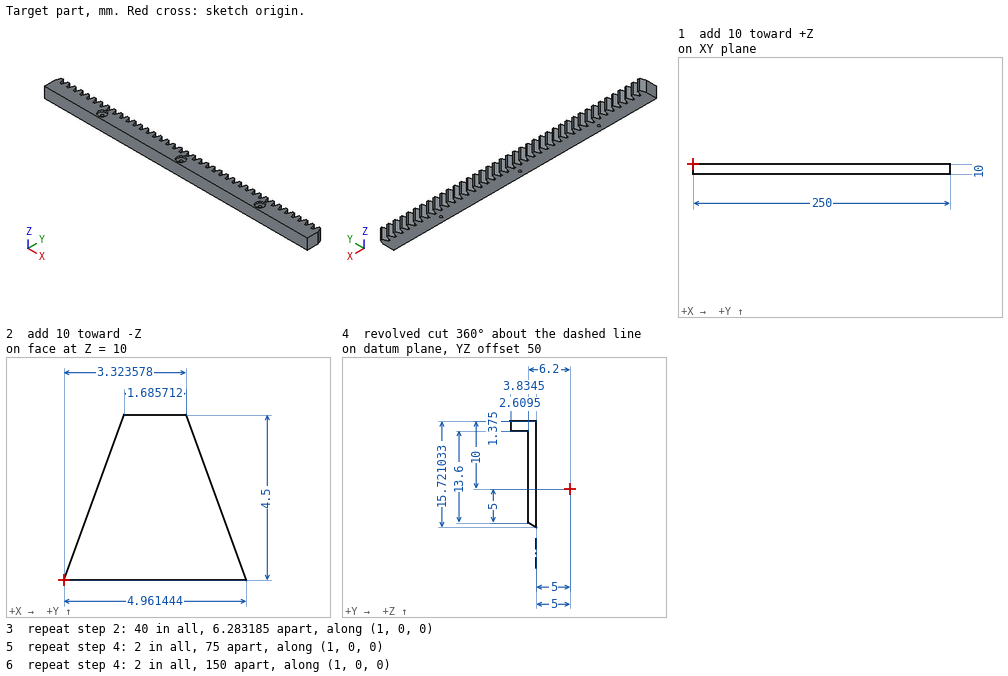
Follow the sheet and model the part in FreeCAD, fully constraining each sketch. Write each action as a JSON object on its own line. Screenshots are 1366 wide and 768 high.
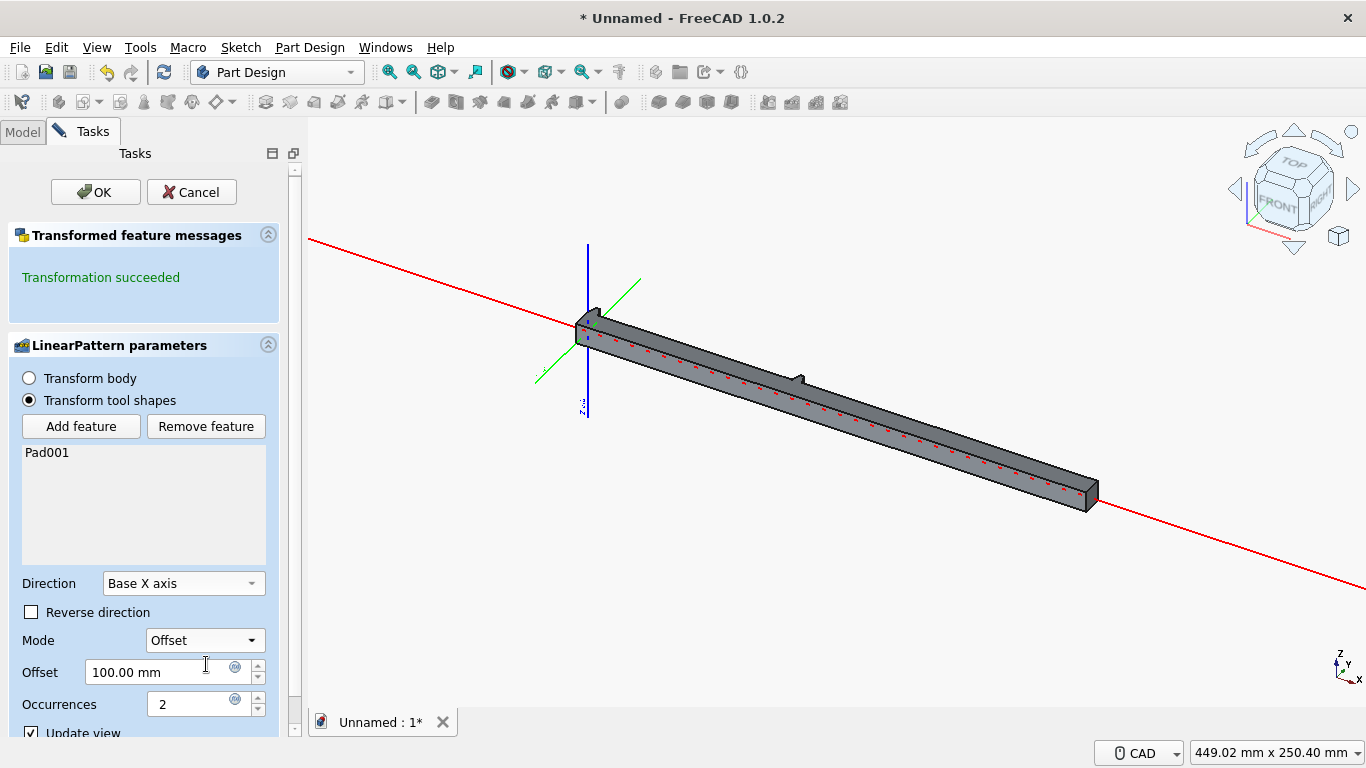
{"action": "triple_click", "coordinate": [168, 672]}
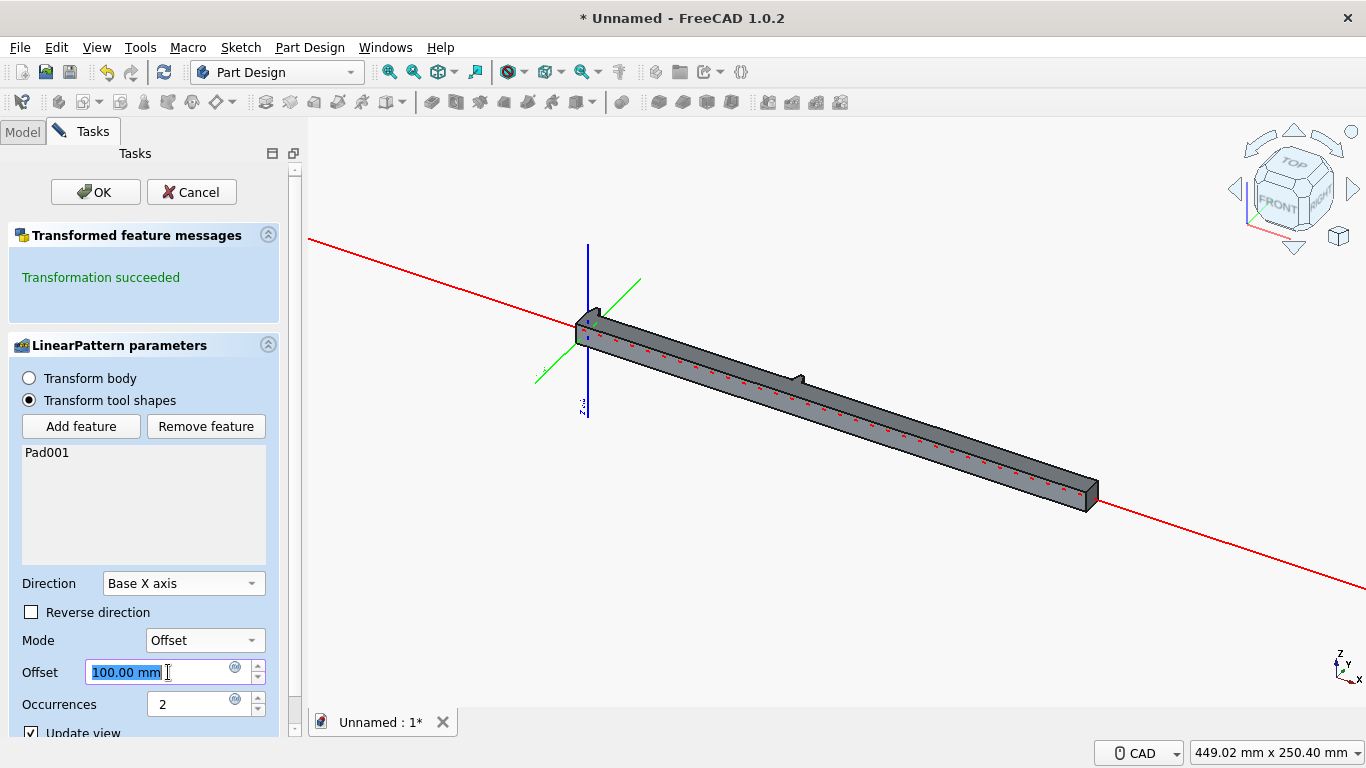
{"action": "type", "text": "6.283185"}
{"action": "key", "text": "Tab"}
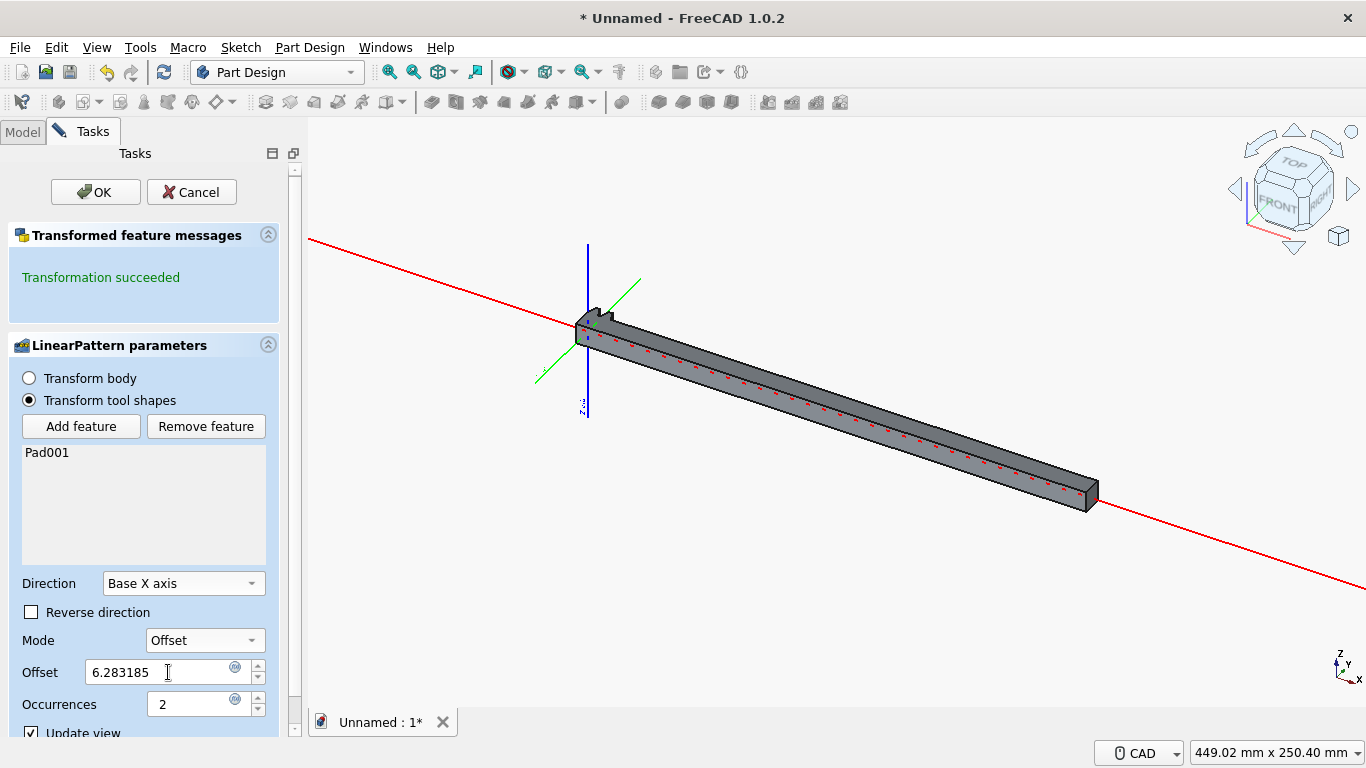
{"action": "triple_click", "coordinate": [198, 704]}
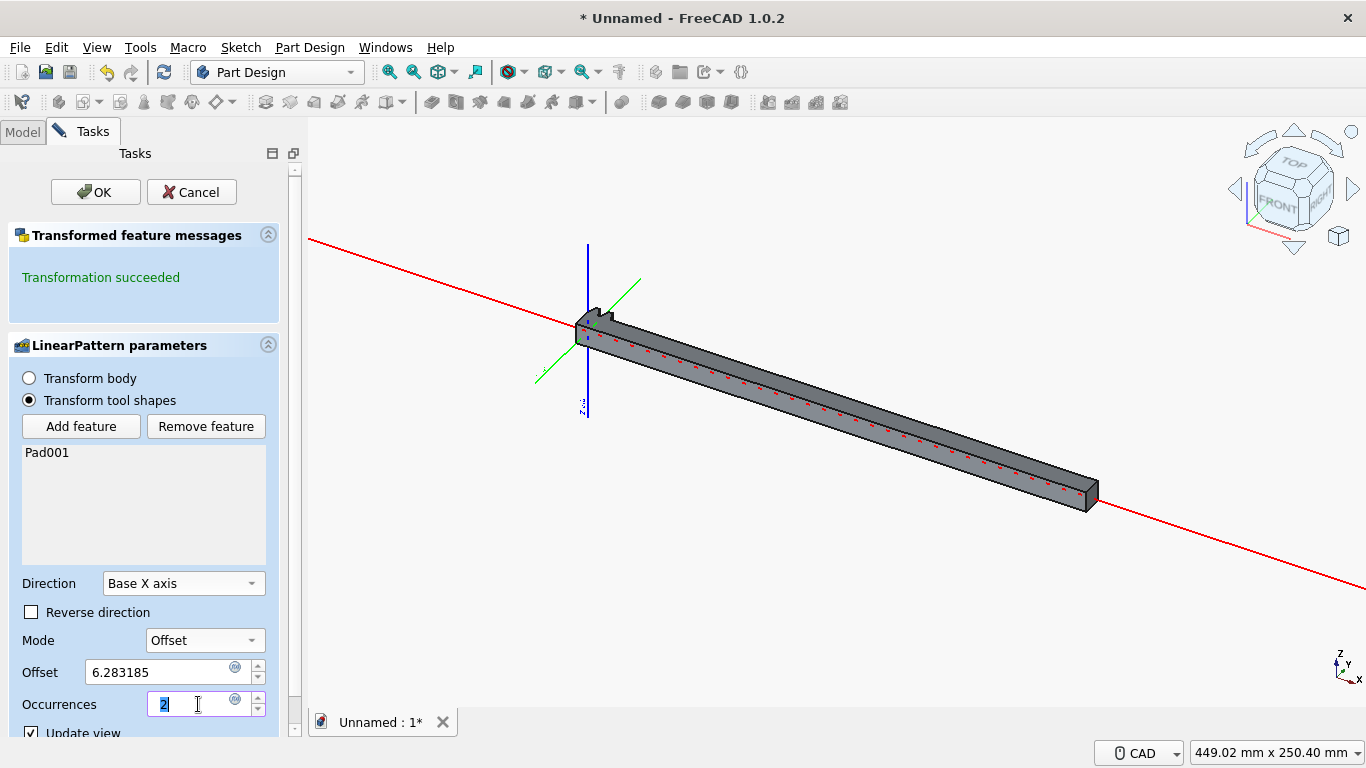
{"action": "type", "text": "40"}
{"action": "key", "text": "Tab"}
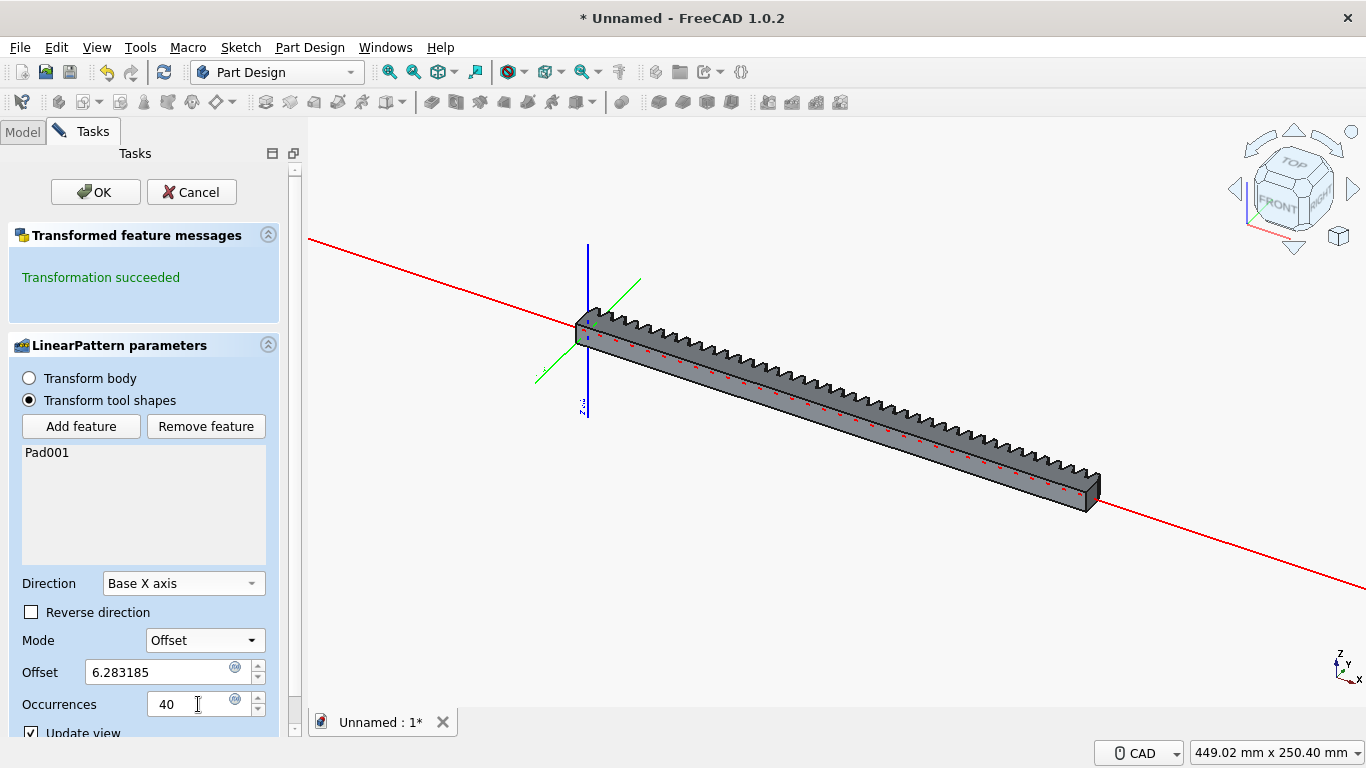
{"action": "left_click", "coordinate": [96, 192]}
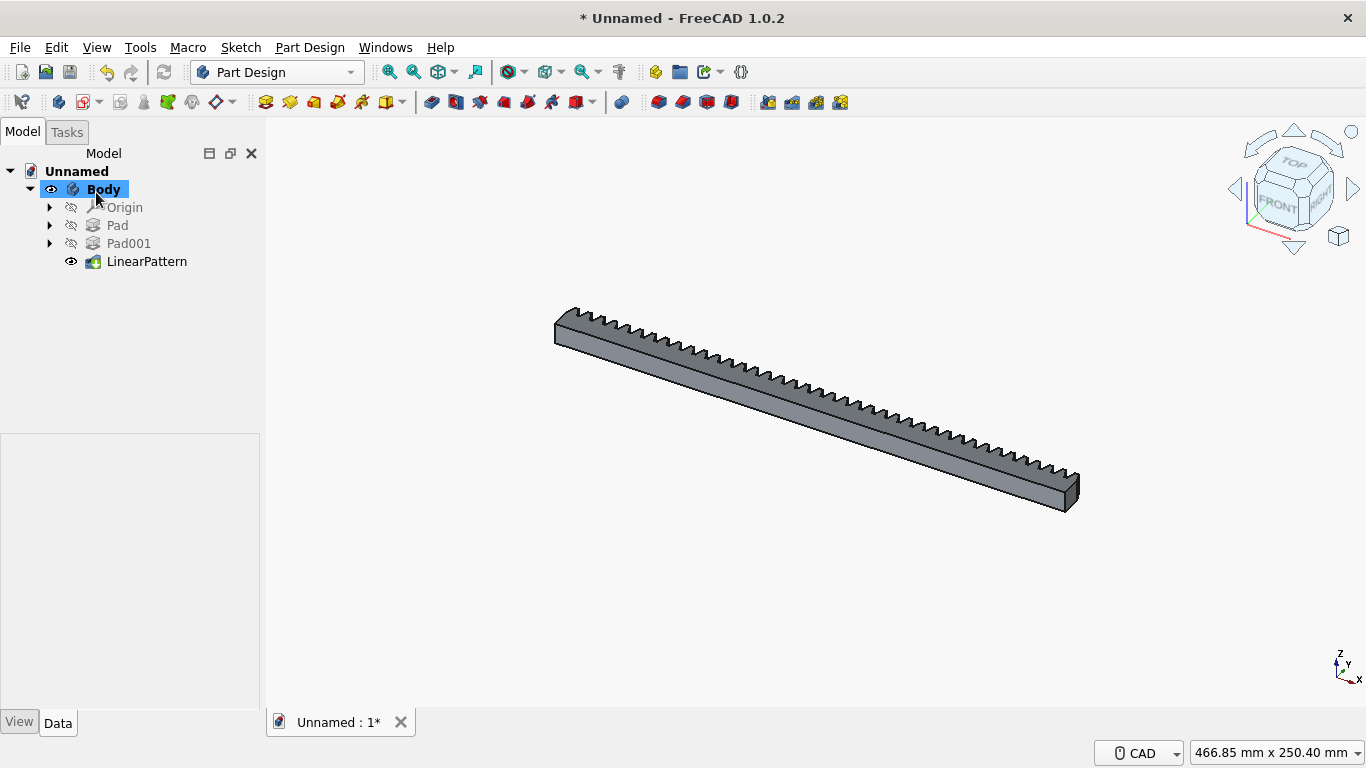
{"action": "left_click", "coordinate": [50, 207]}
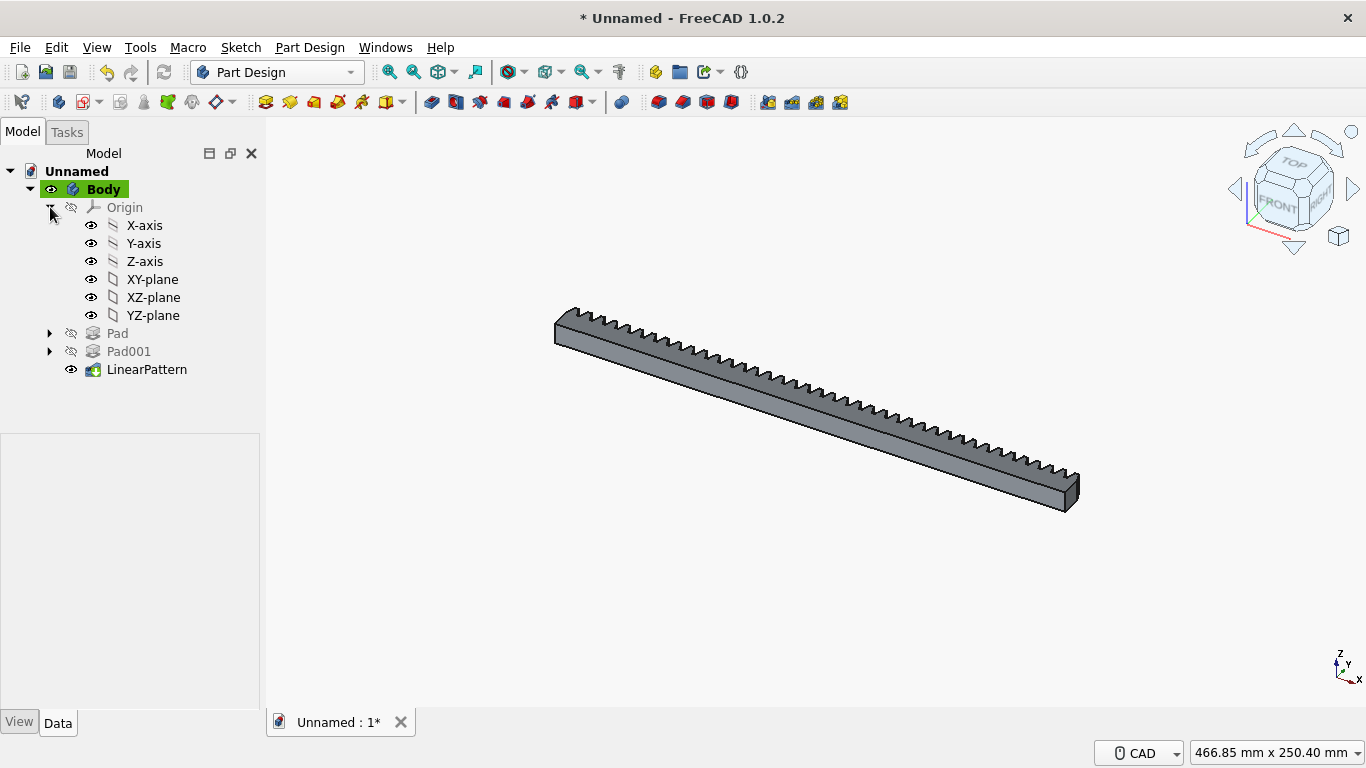
{"action": "left_click", "coordinate": [136, 315]}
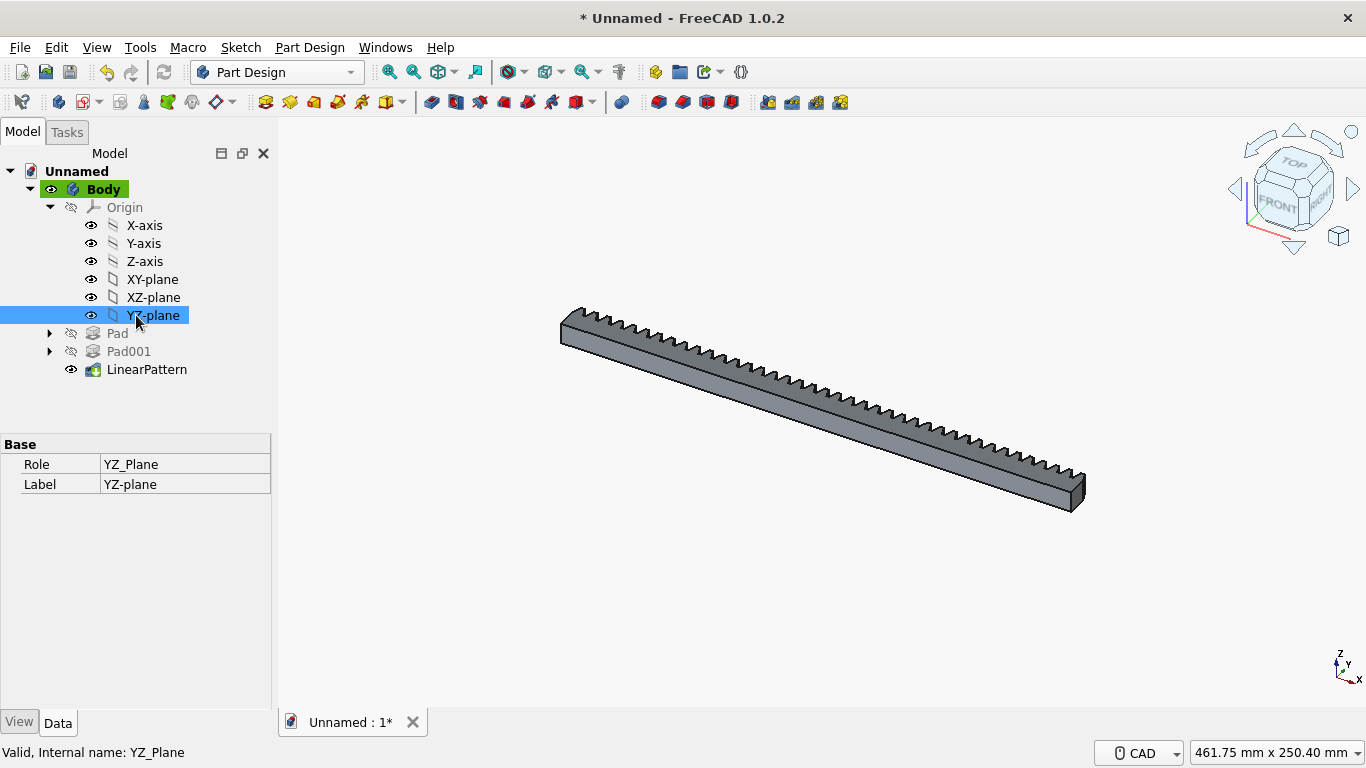
{"action": "left_click", "coordinate": [216, 102]}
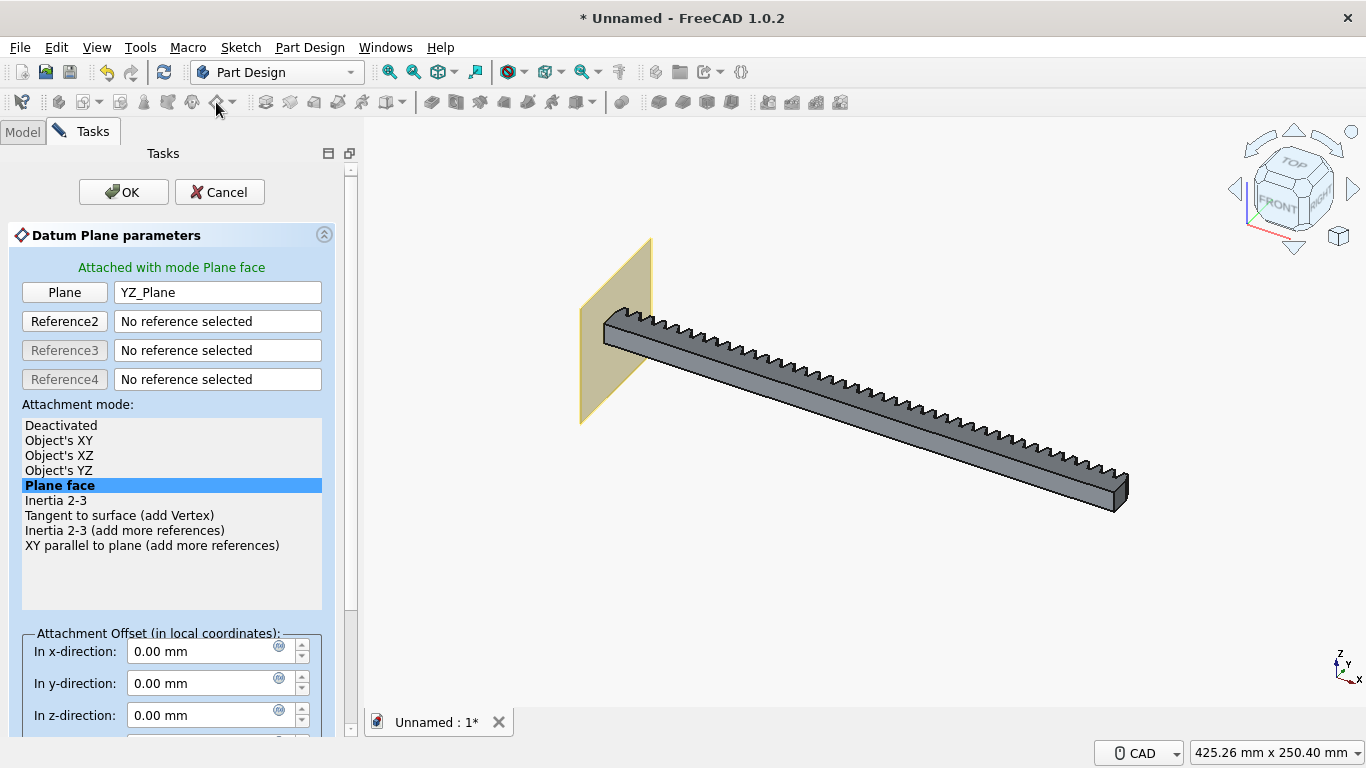
{"action": "triple_click", "coordinate": [210, 715]}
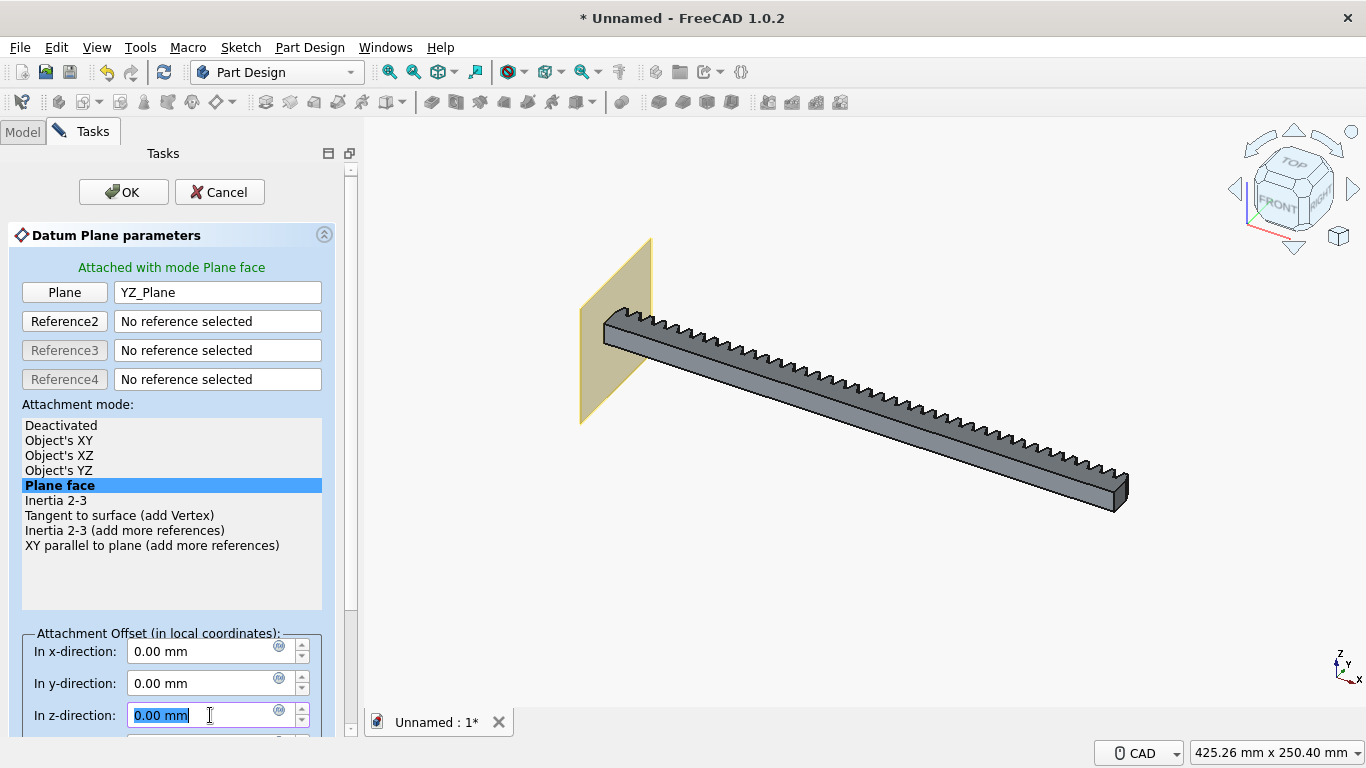
{"action": "type", "text": "50"}
{"action": "key", "text": "Tab"}